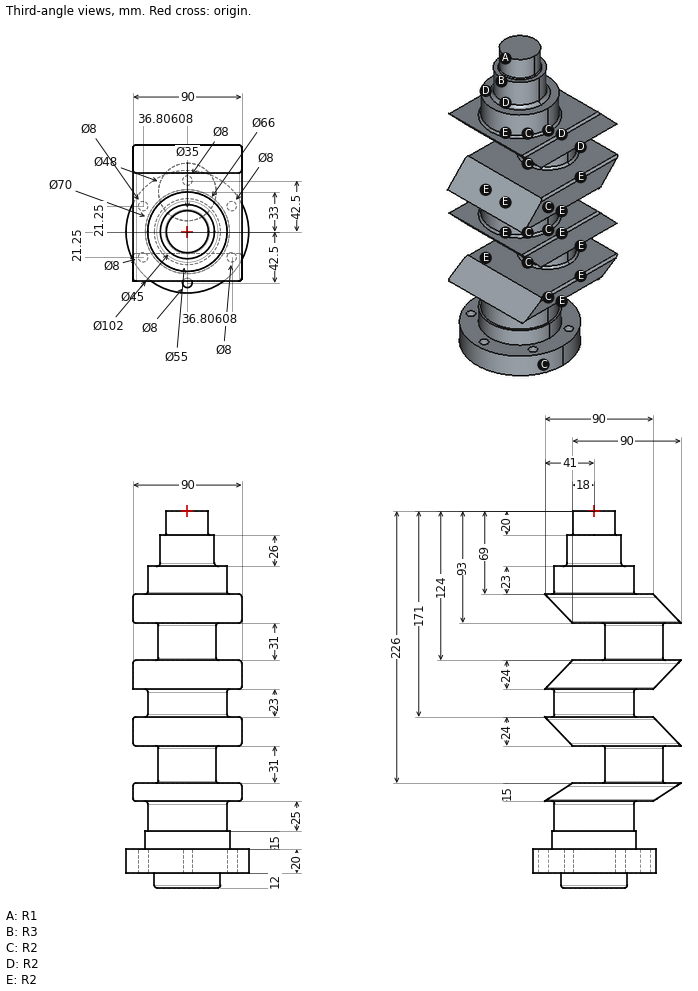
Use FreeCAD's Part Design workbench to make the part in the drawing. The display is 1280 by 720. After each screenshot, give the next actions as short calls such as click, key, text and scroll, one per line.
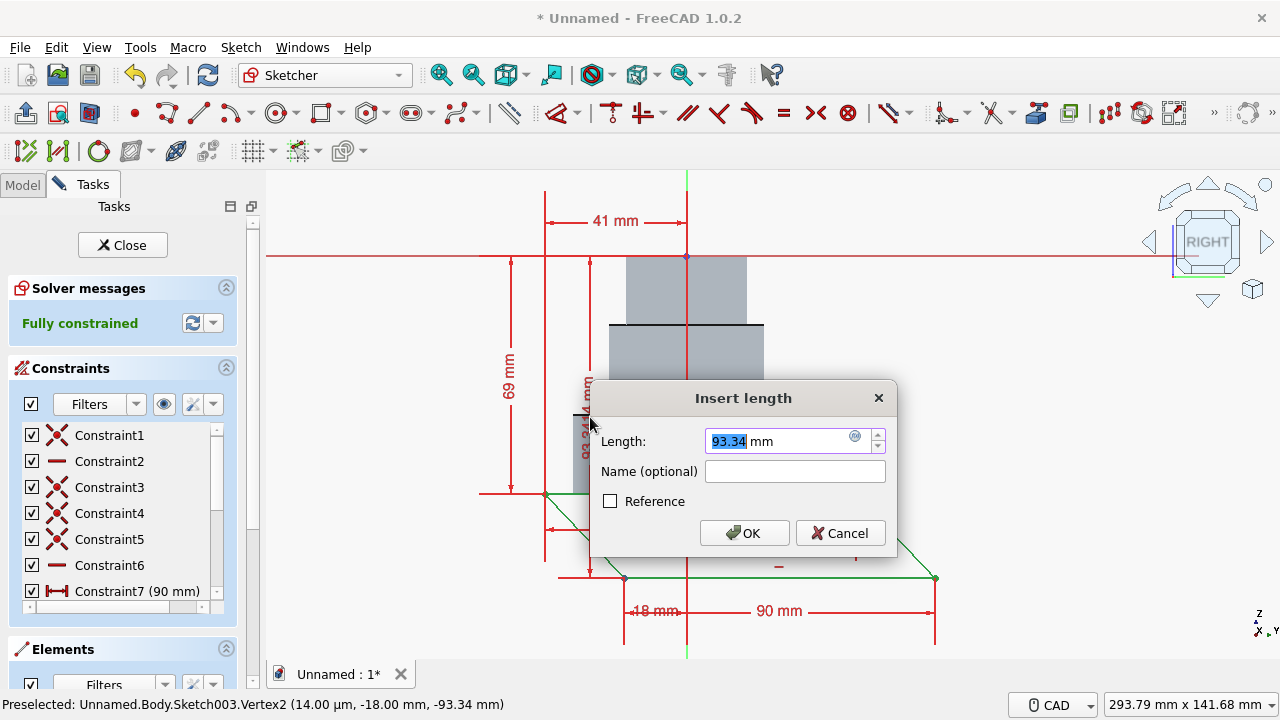
text(93)
key(Return)
key(Escape)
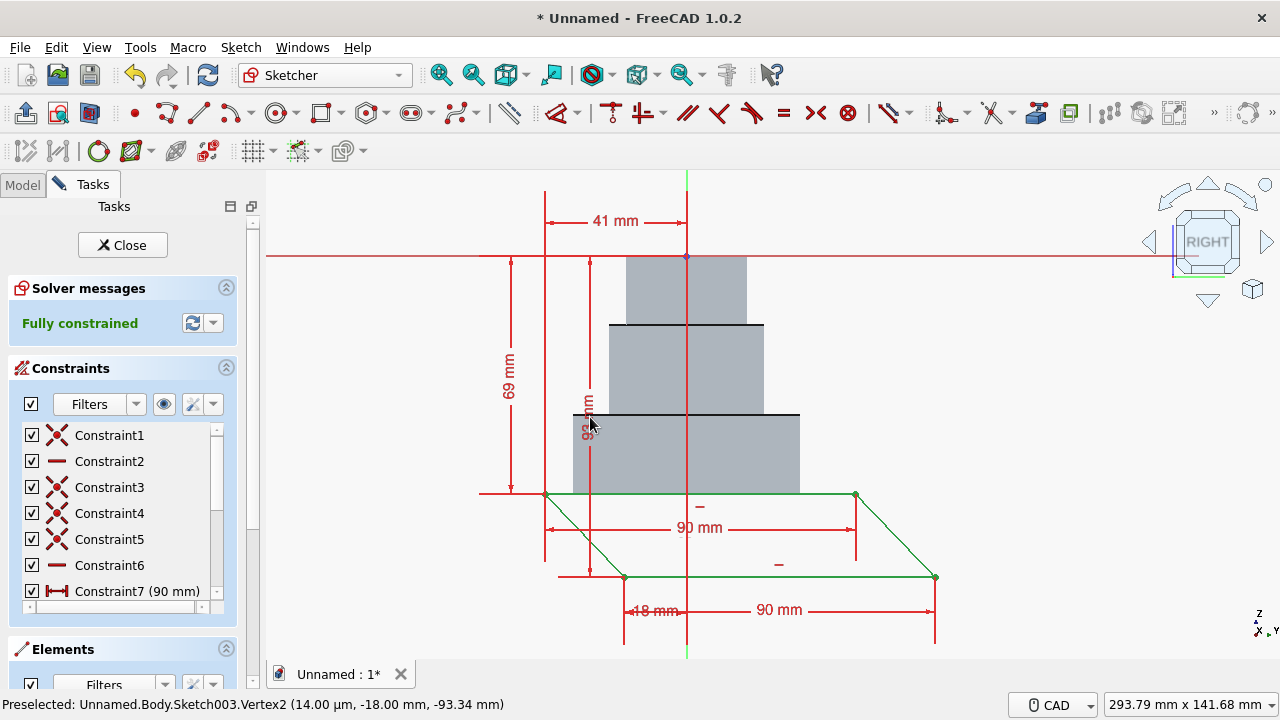
click(123, 245)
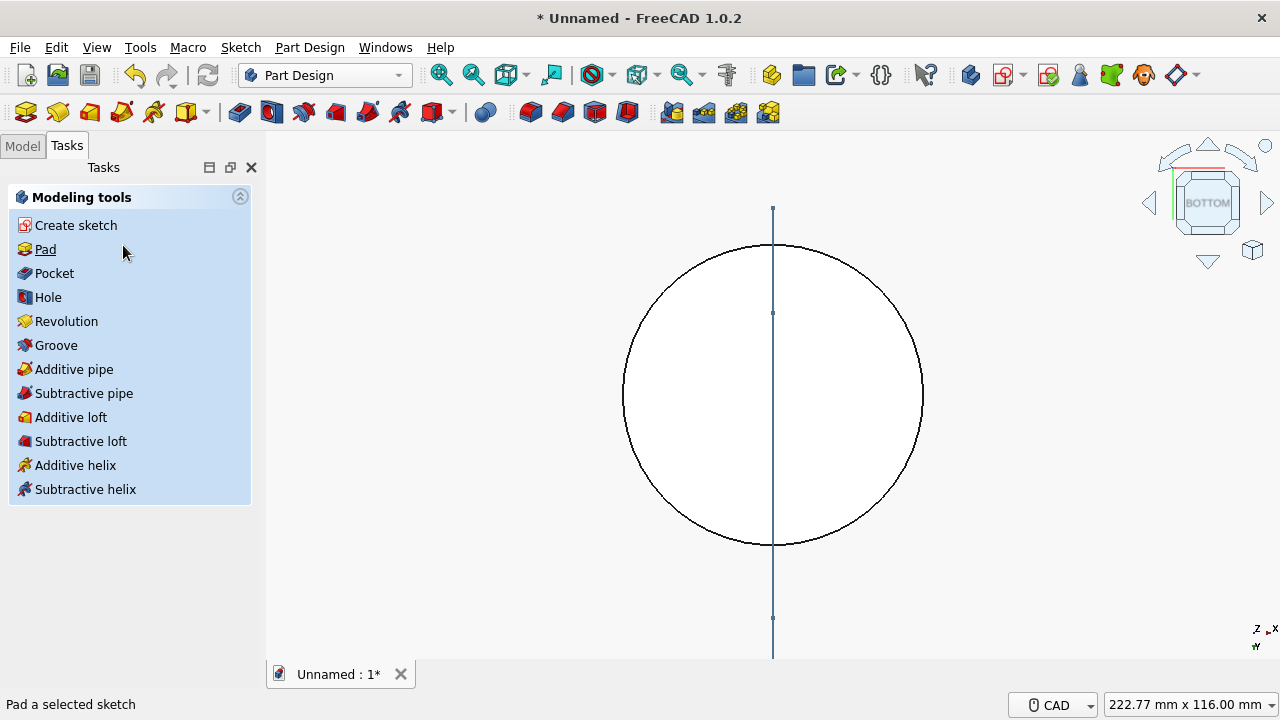
click(26, 112)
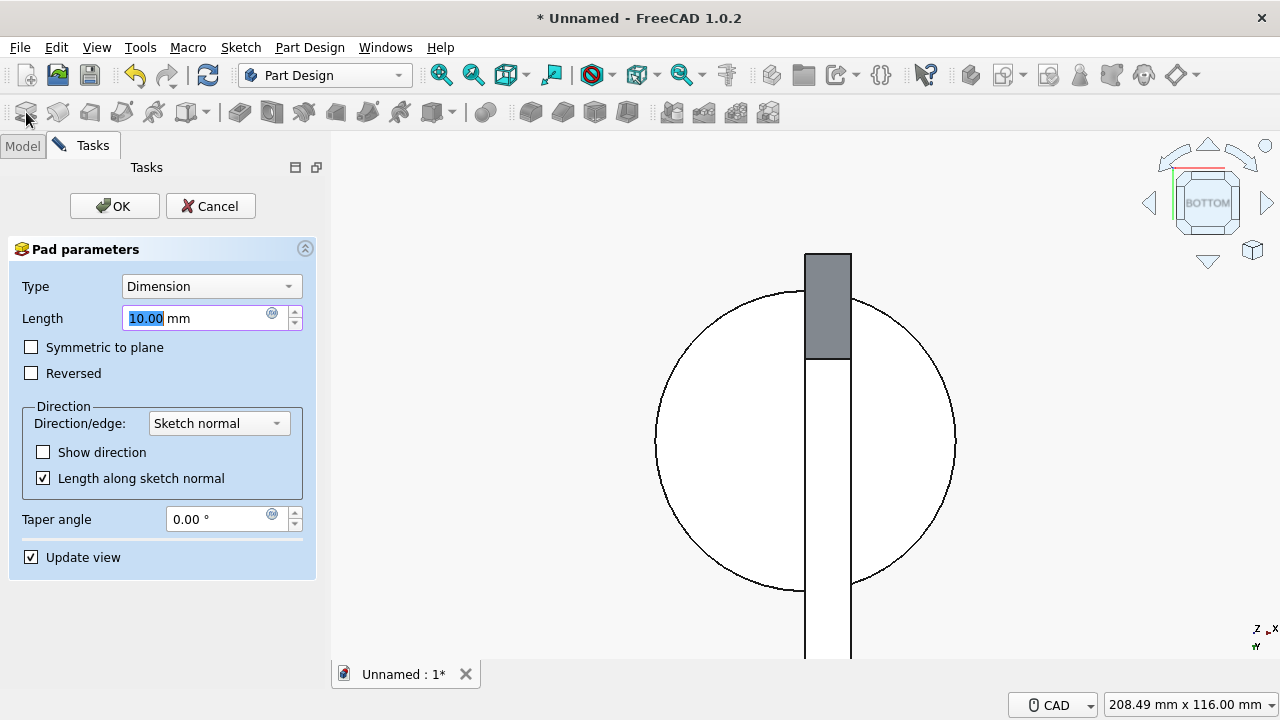
text(90)
key(Tab)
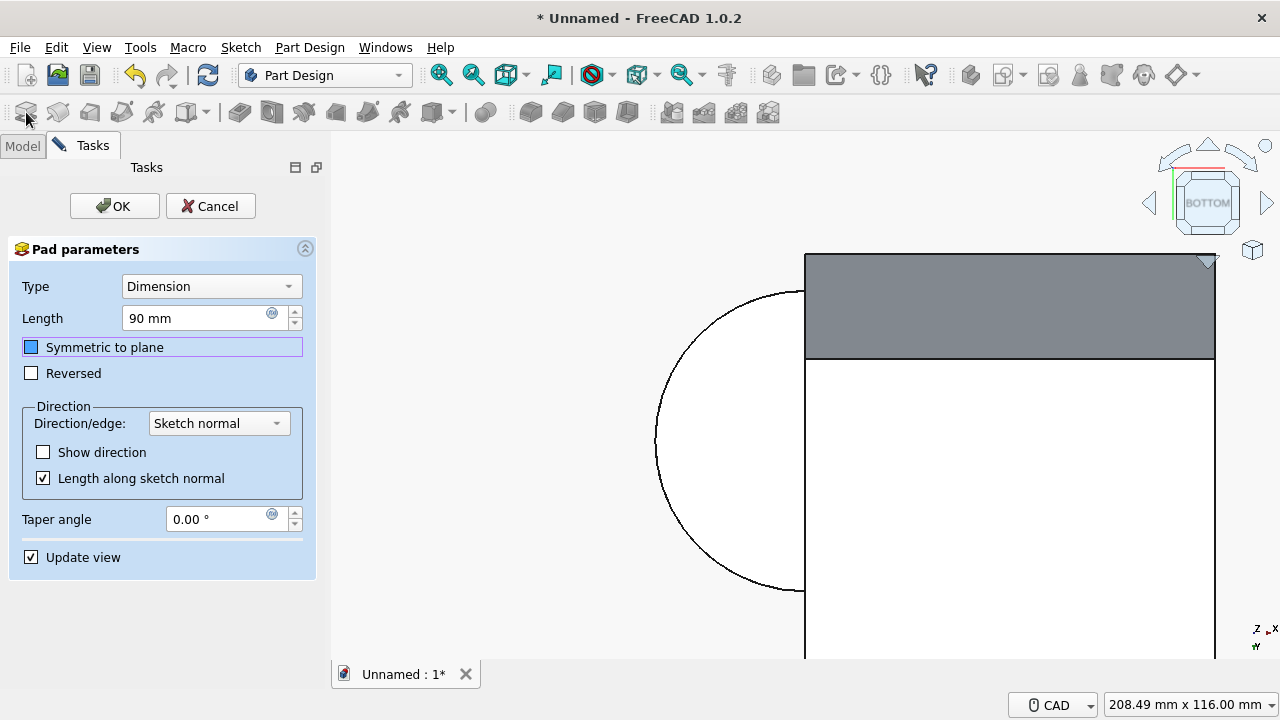
click(30, 347)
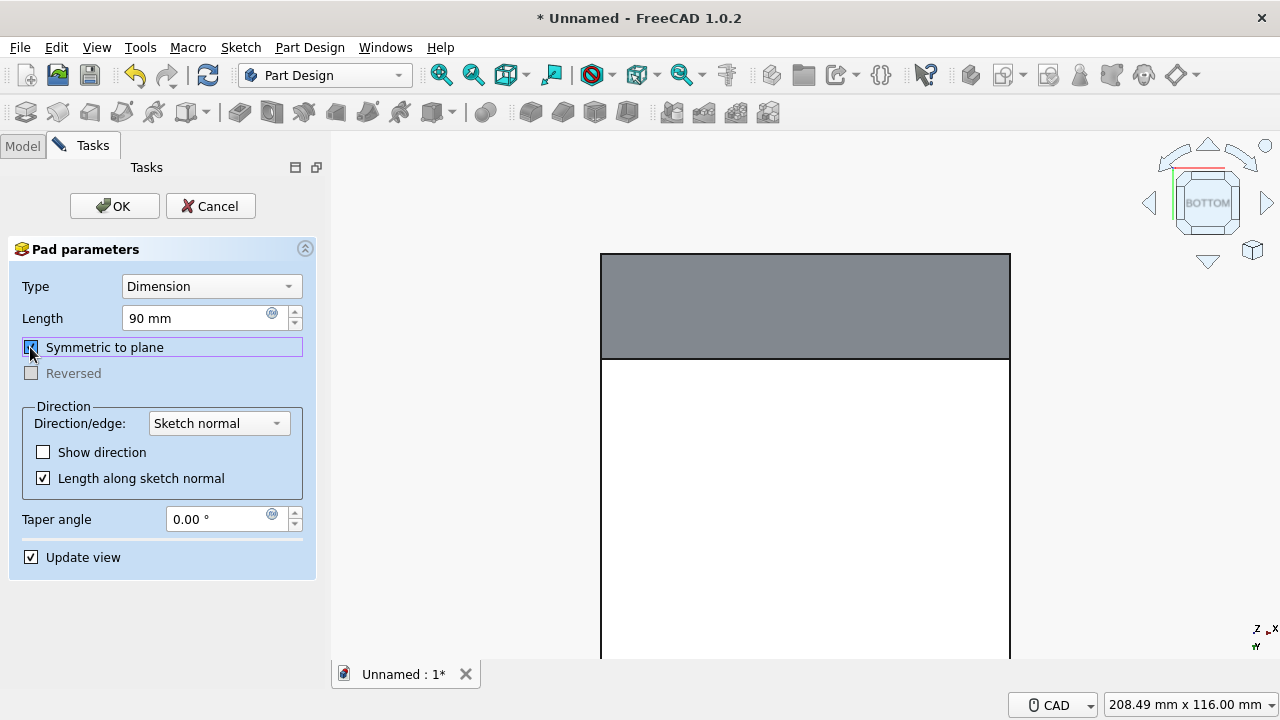
click(115, 206)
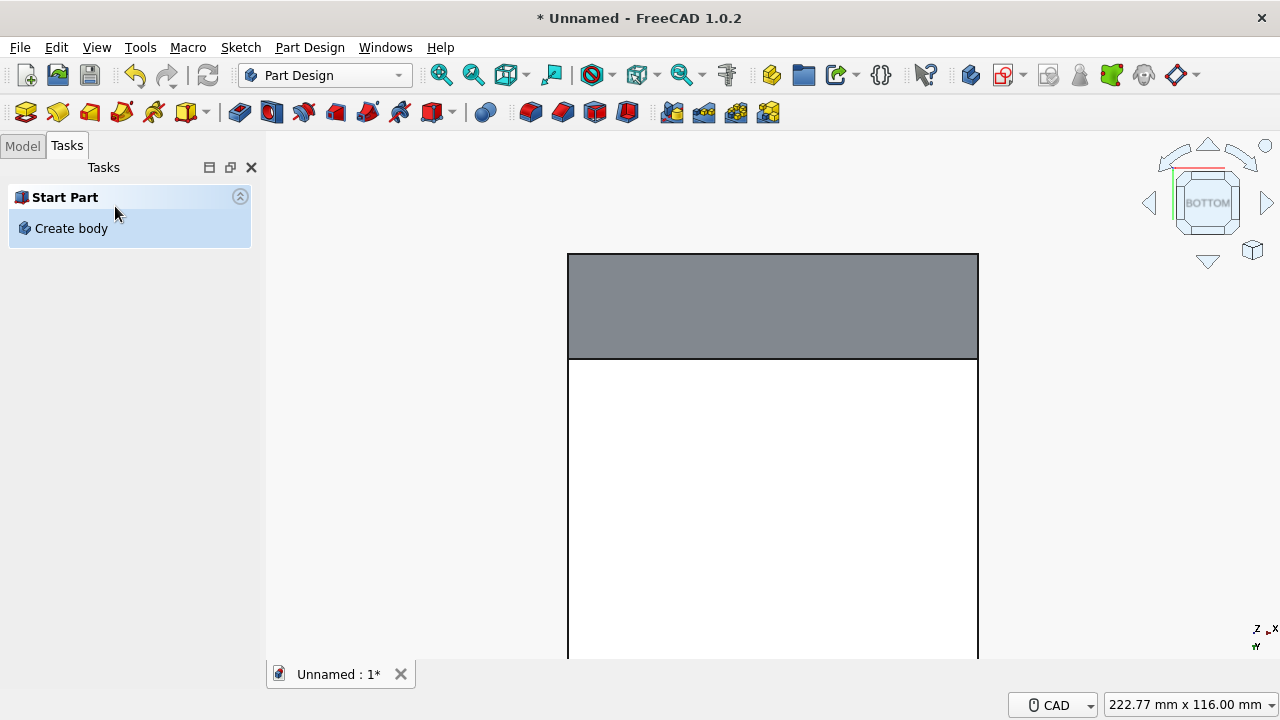
click(442, 76)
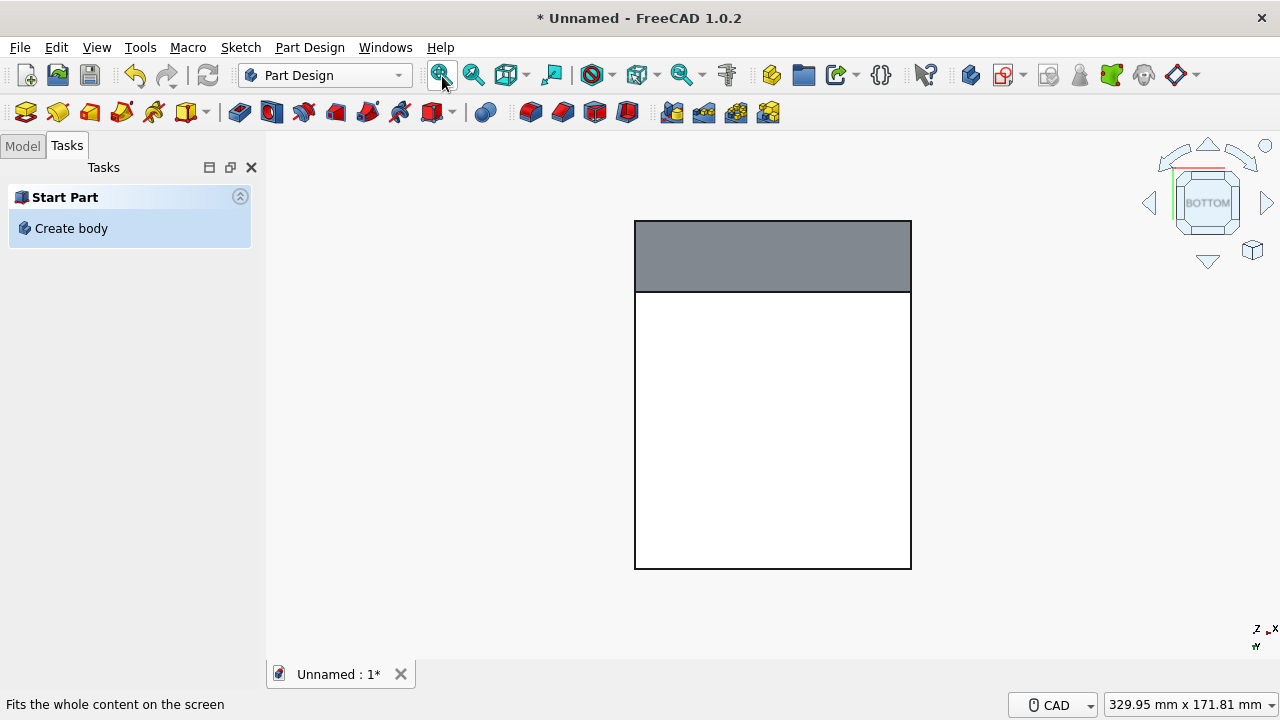
click(773, 429)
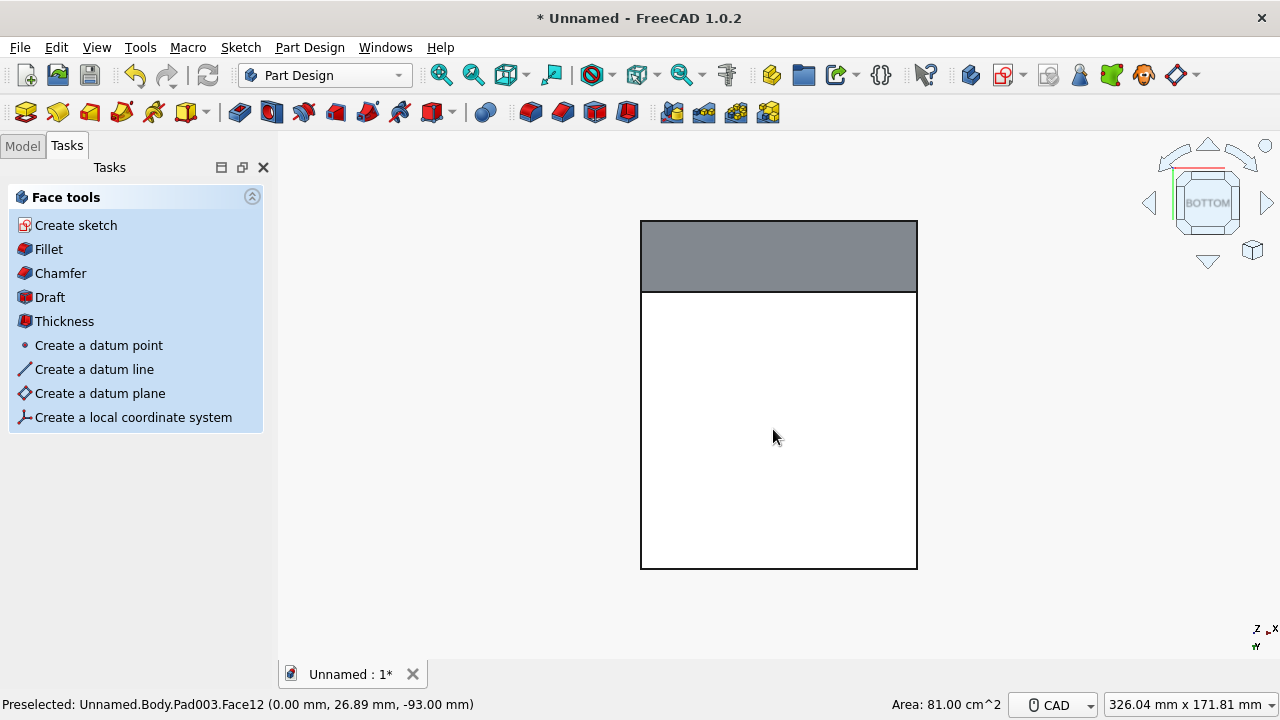
click(1004, 76)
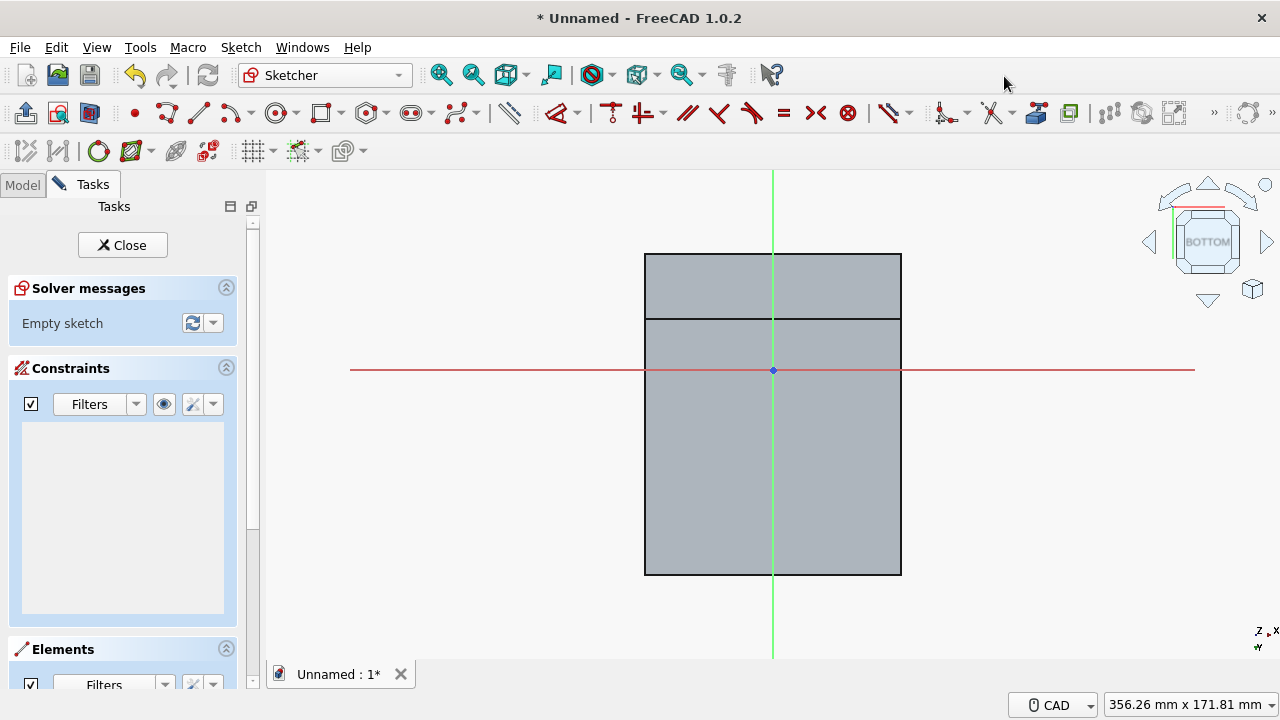
scroll(856, 497, up, 3)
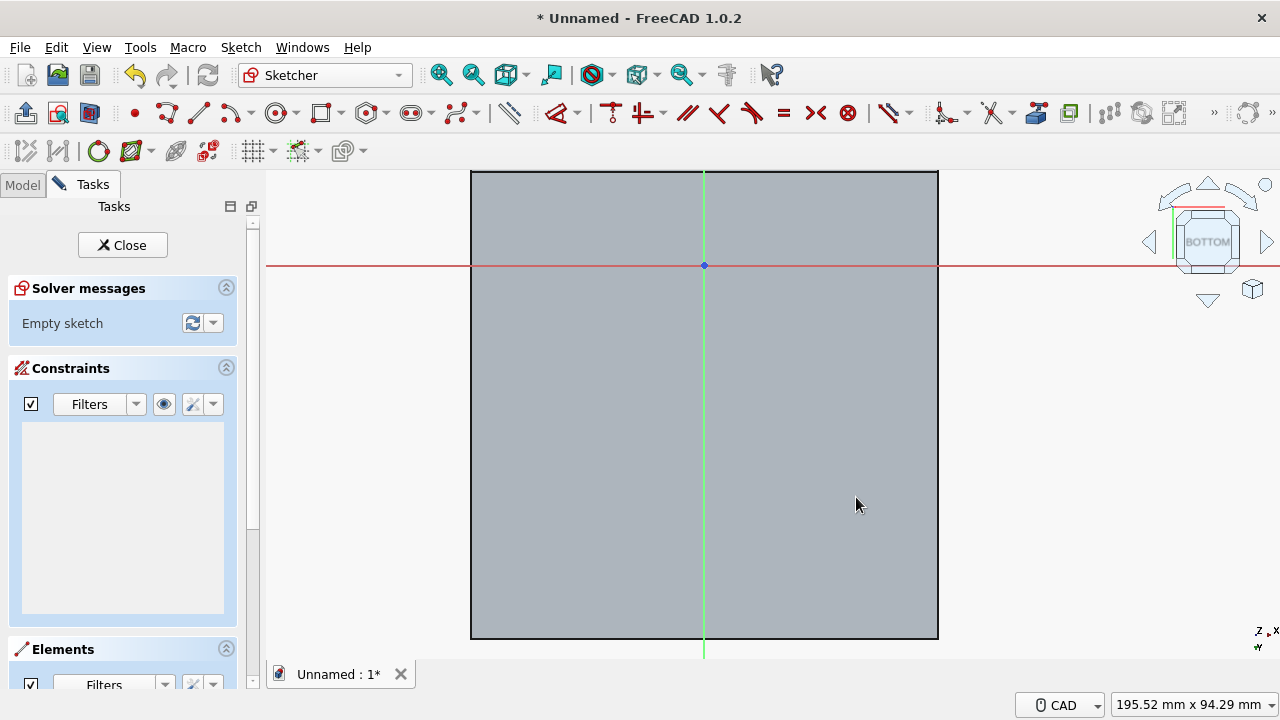
click(276, 114)